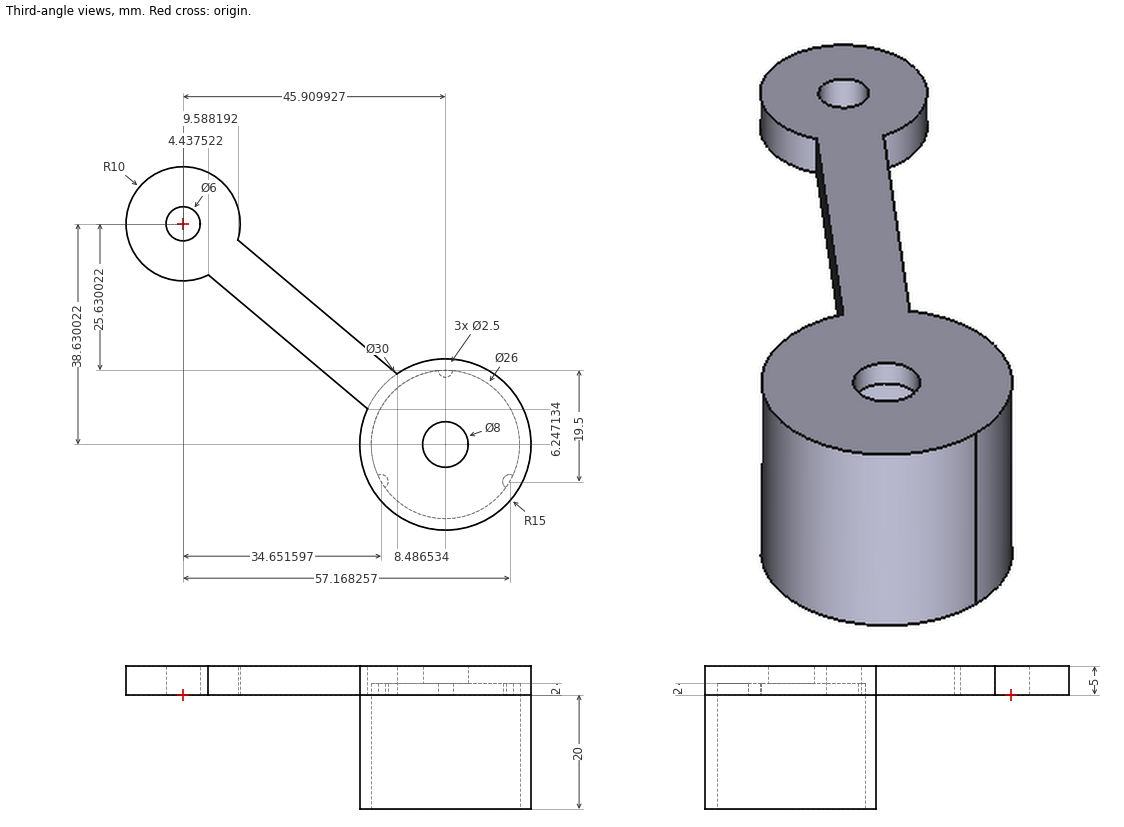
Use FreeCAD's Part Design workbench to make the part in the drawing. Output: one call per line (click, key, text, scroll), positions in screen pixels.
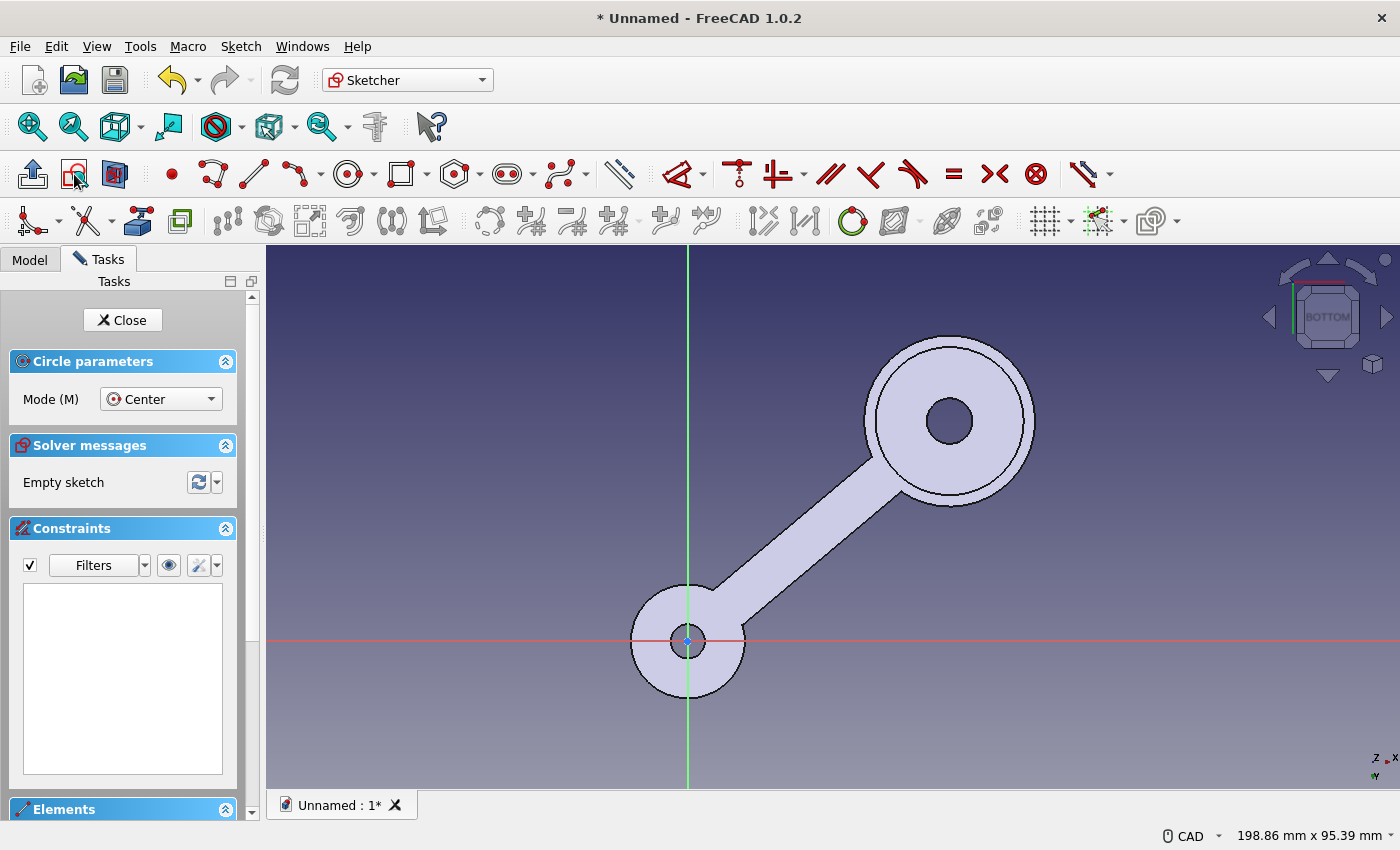
scroll(950, 495, up, 6)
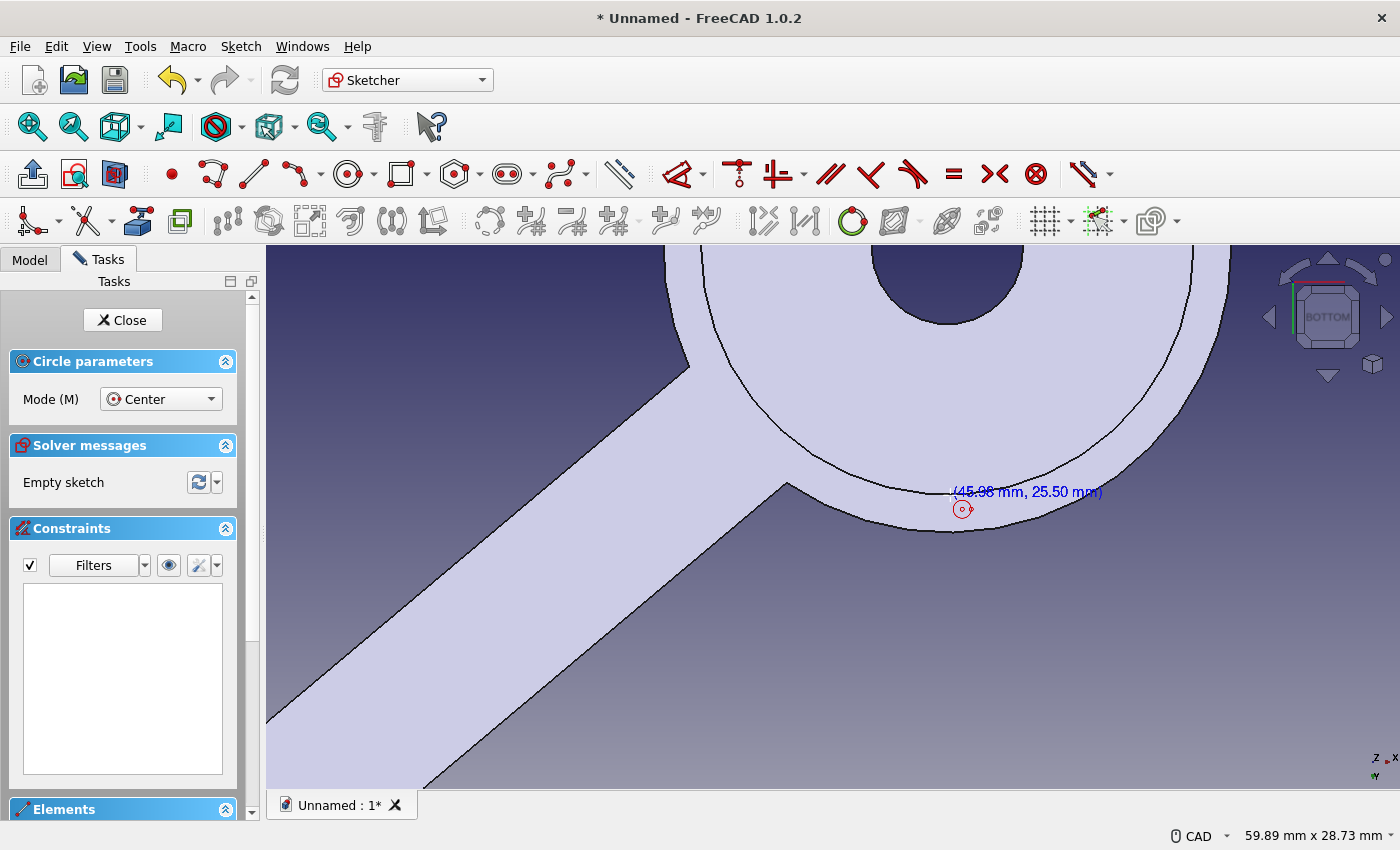
click(947, 495)
move(964, 478)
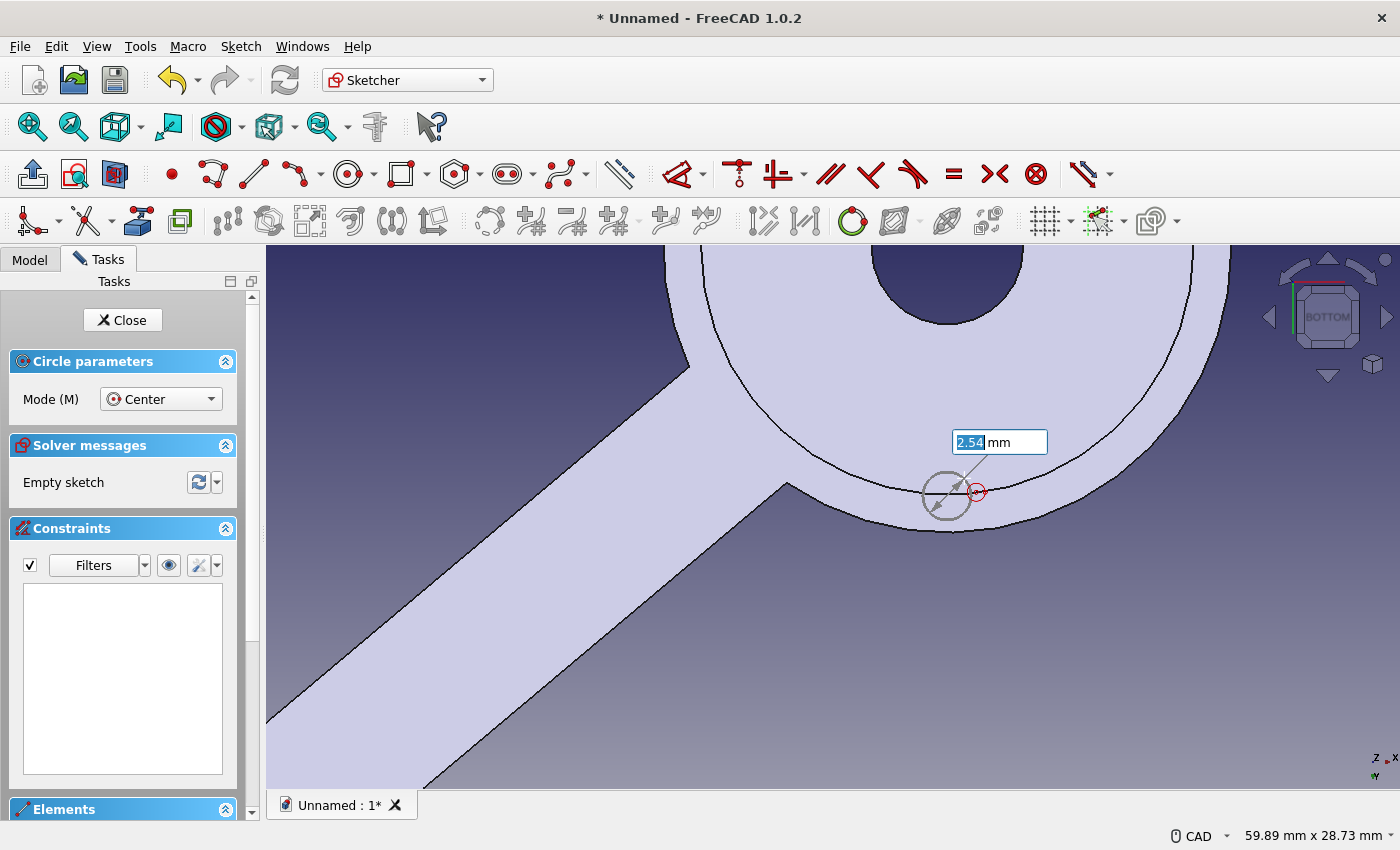
text(2.5)
key(Return)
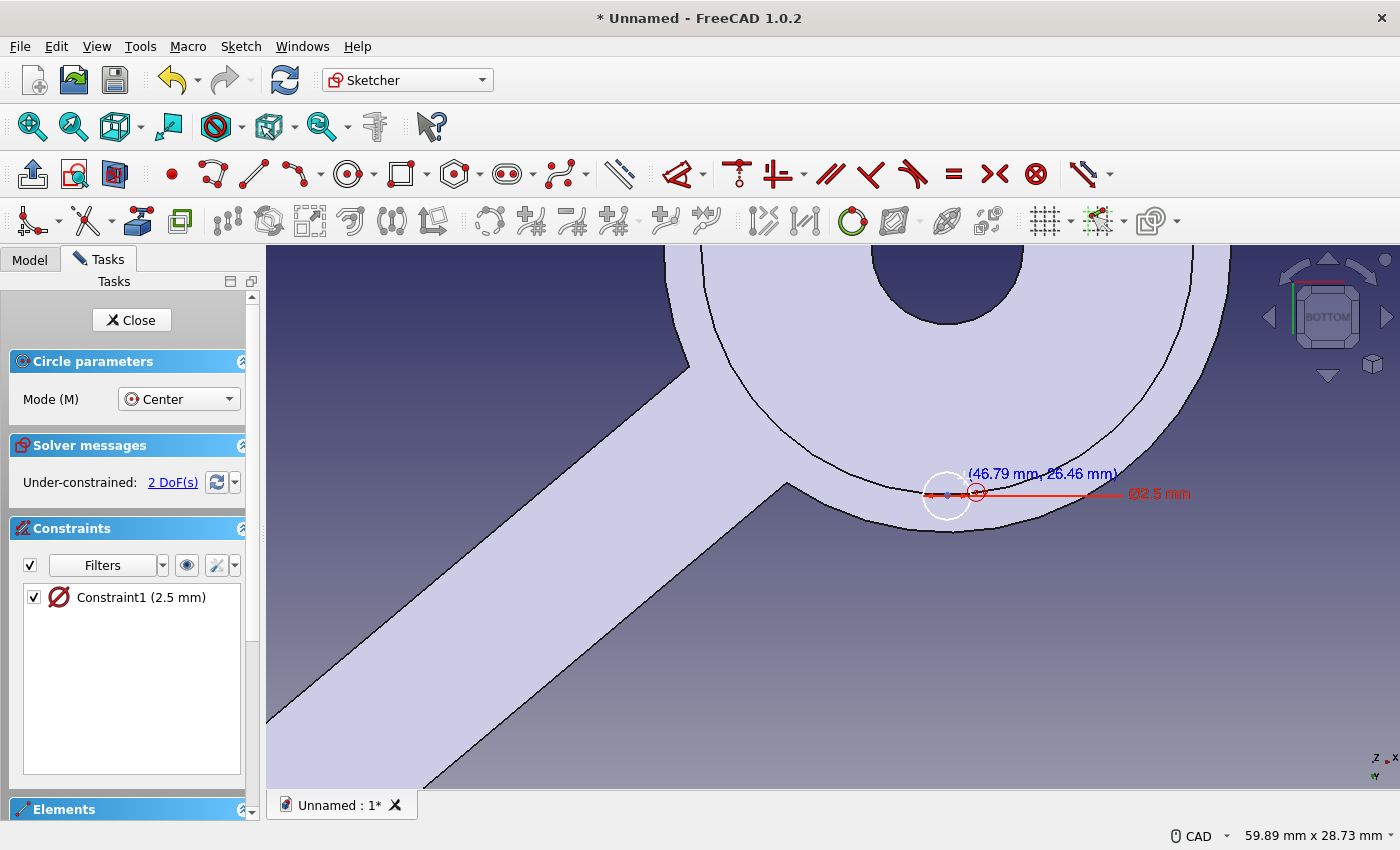
scroll(842, 503, down, 5)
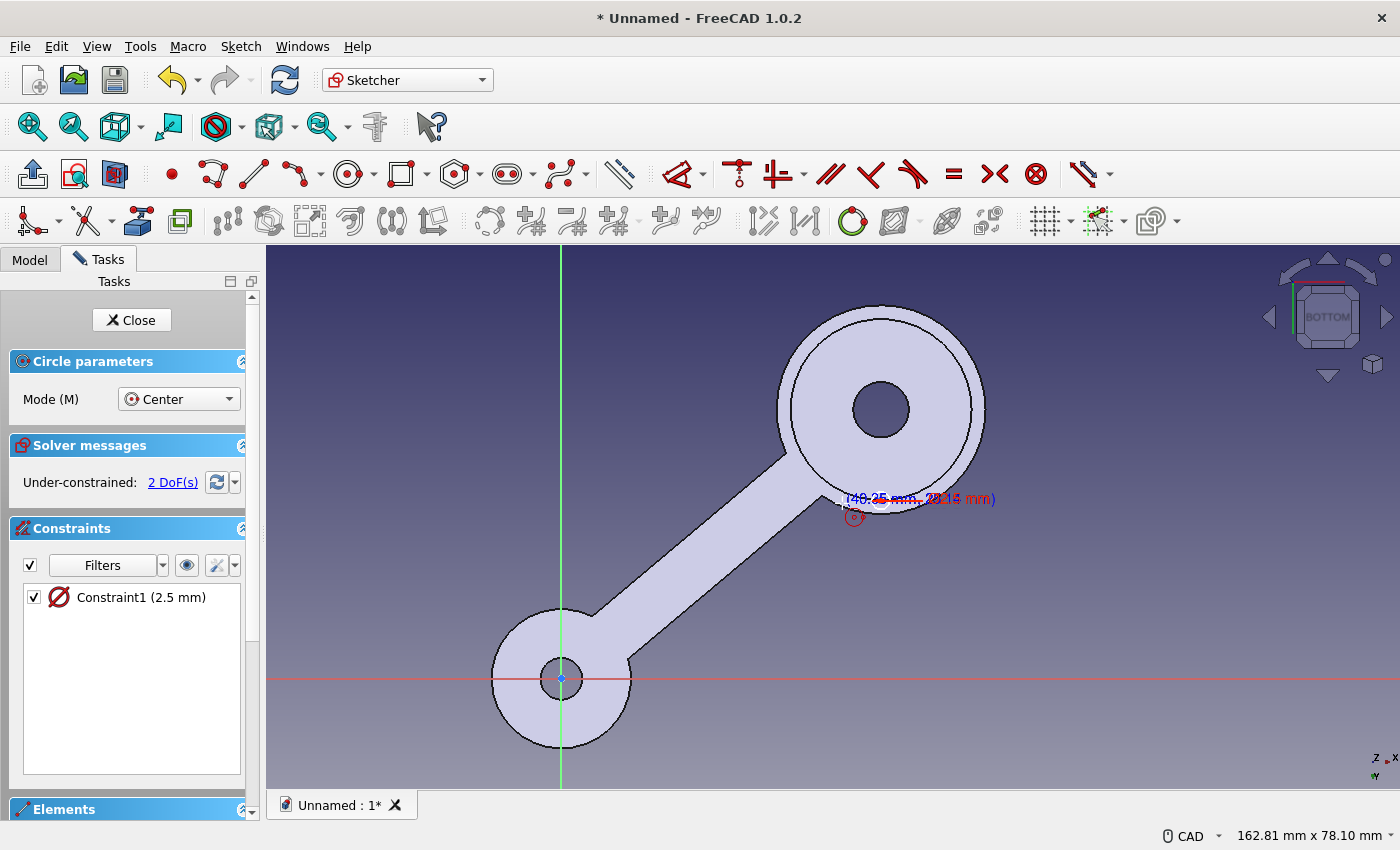
scroll(959, 364, up, 5)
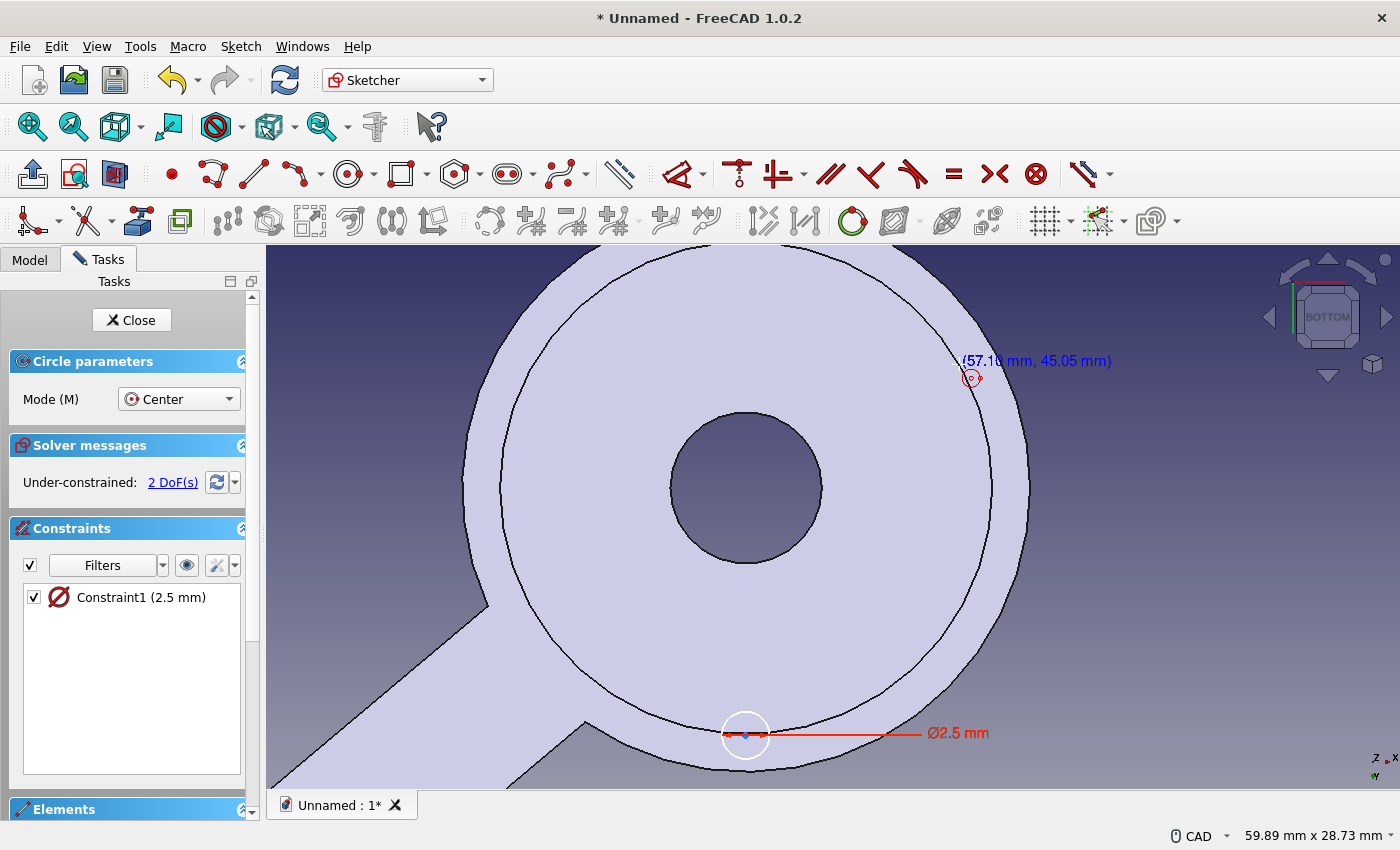
click(959, 365)
move(976, 348)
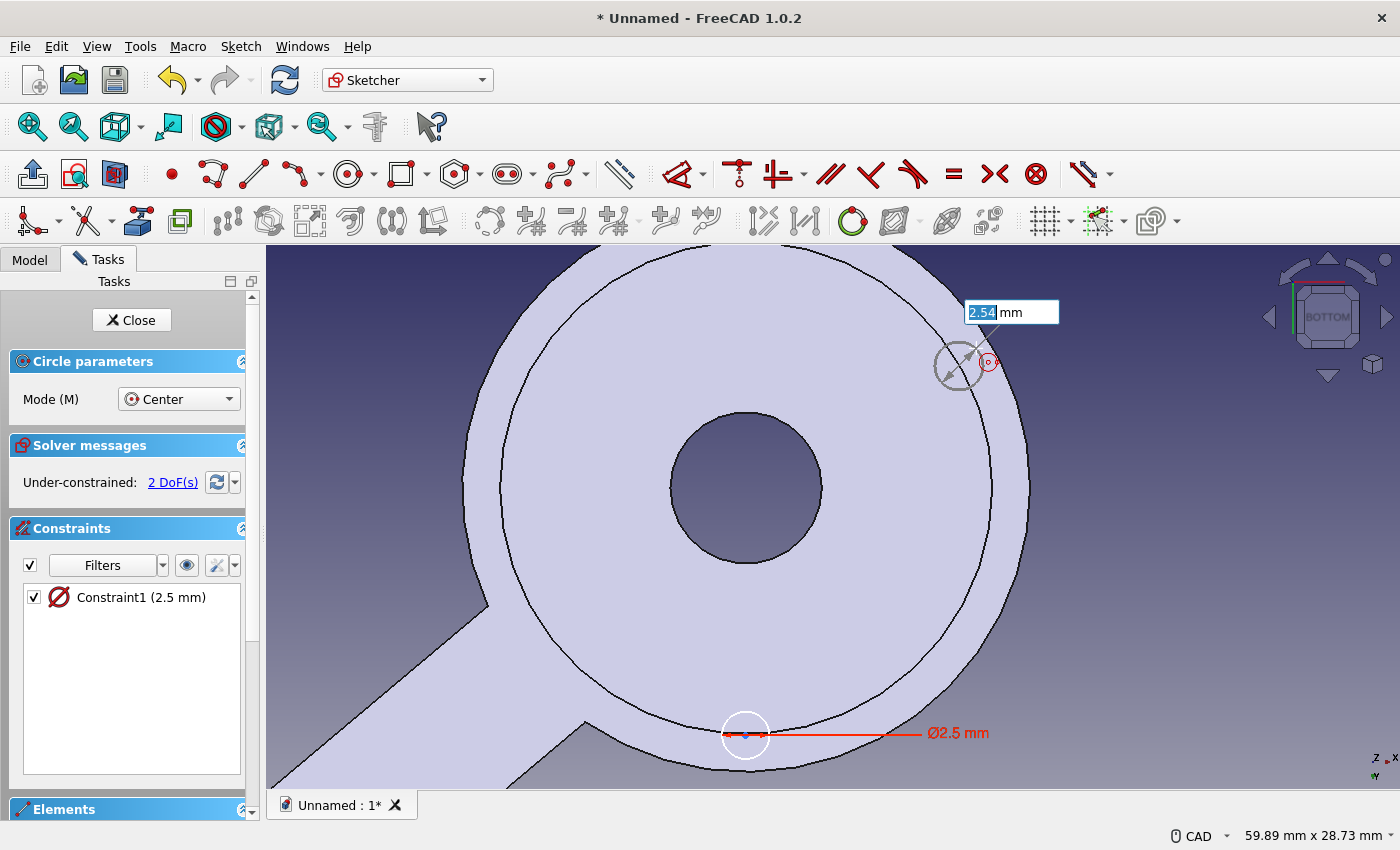
text(2.5)
key(Return)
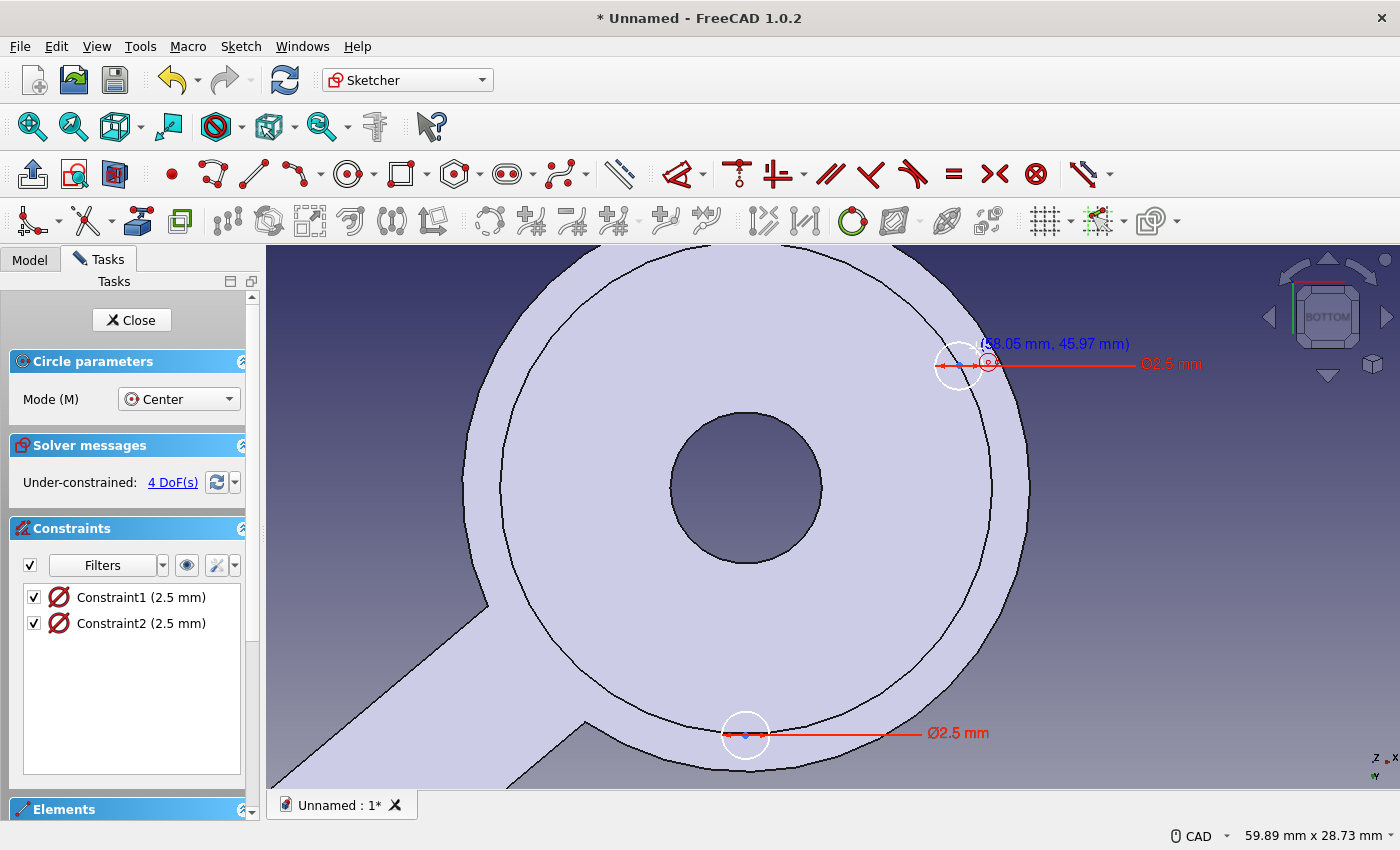
click(533, 365)
move(550, 348)